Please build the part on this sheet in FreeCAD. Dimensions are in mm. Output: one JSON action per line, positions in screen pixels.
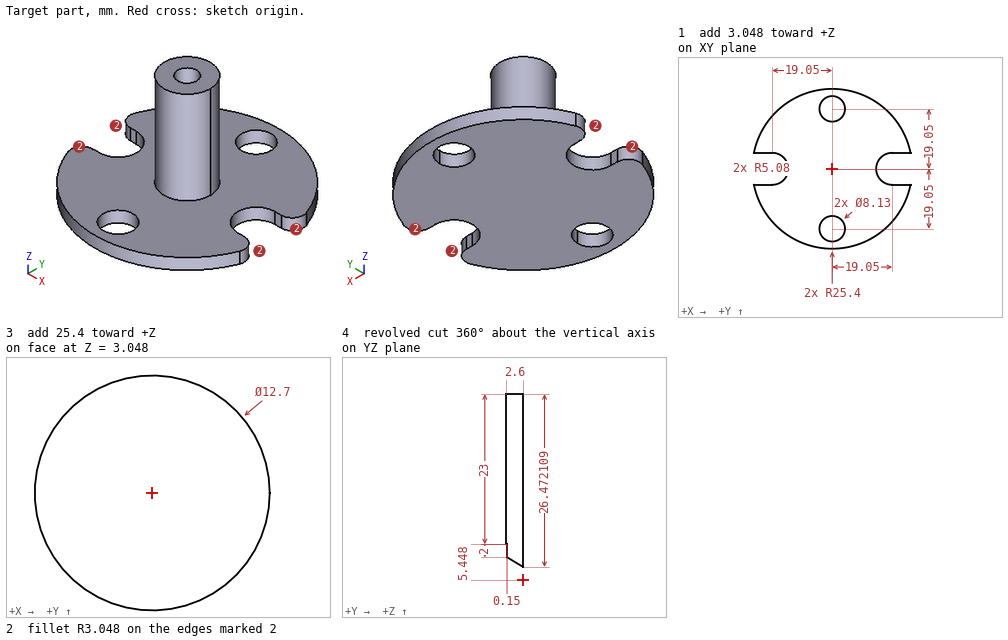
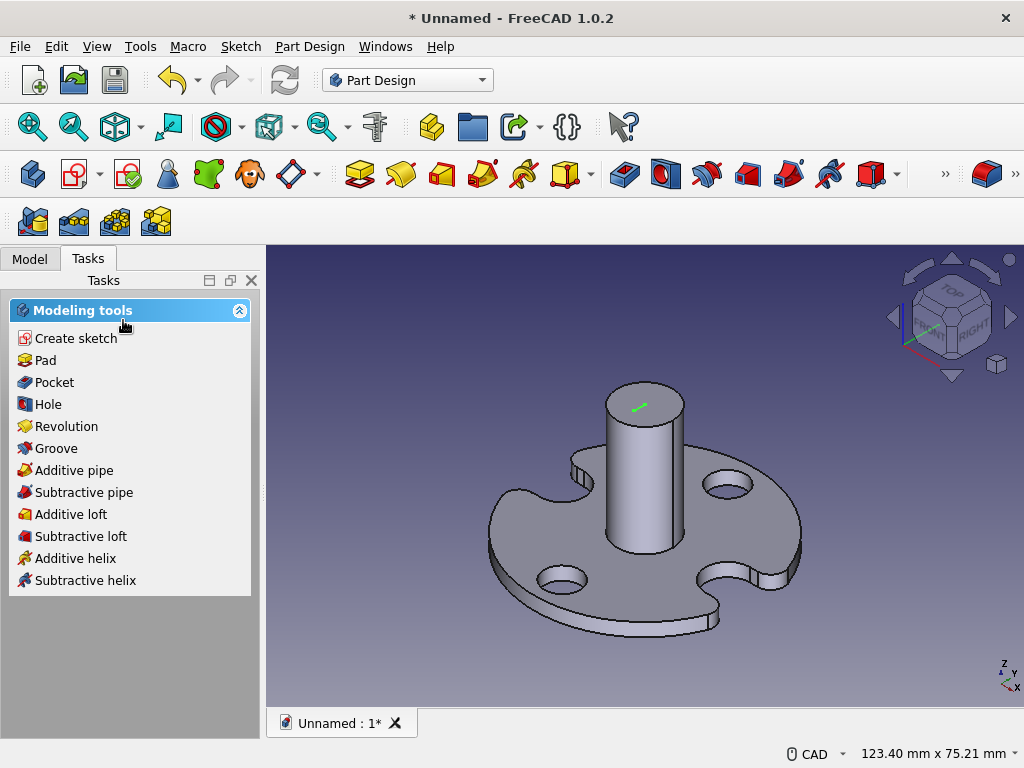
{"action": "left_click", "coordinate": [707, 174]}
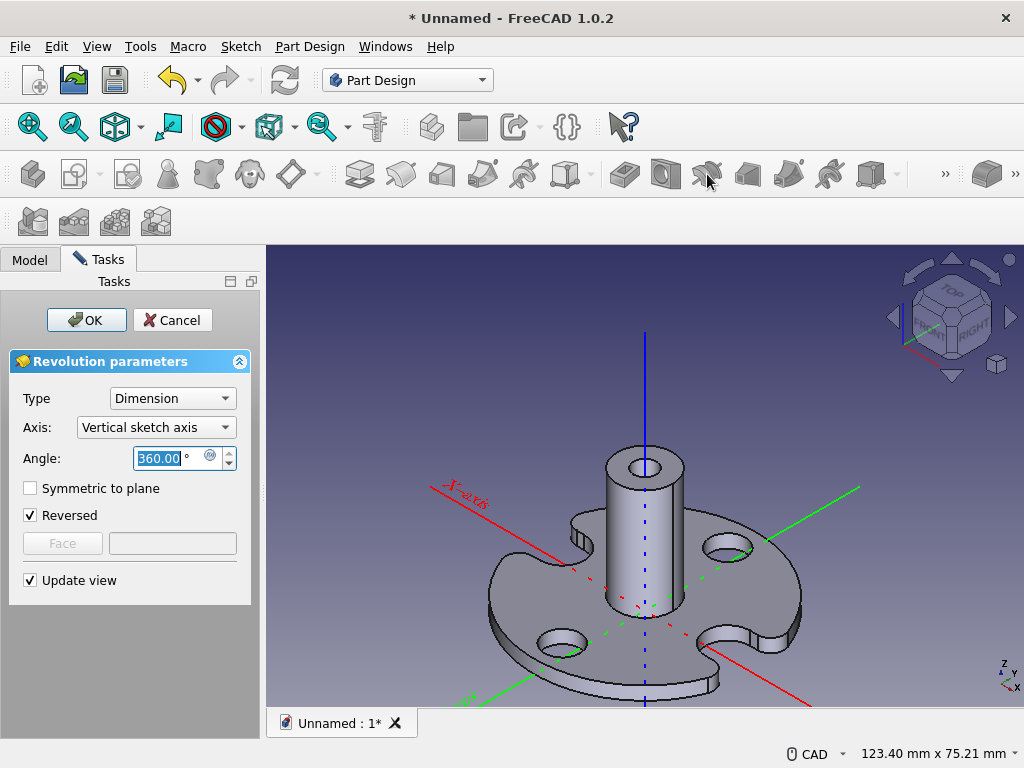
{"action": "left_click", "coordinate": [87, 320]}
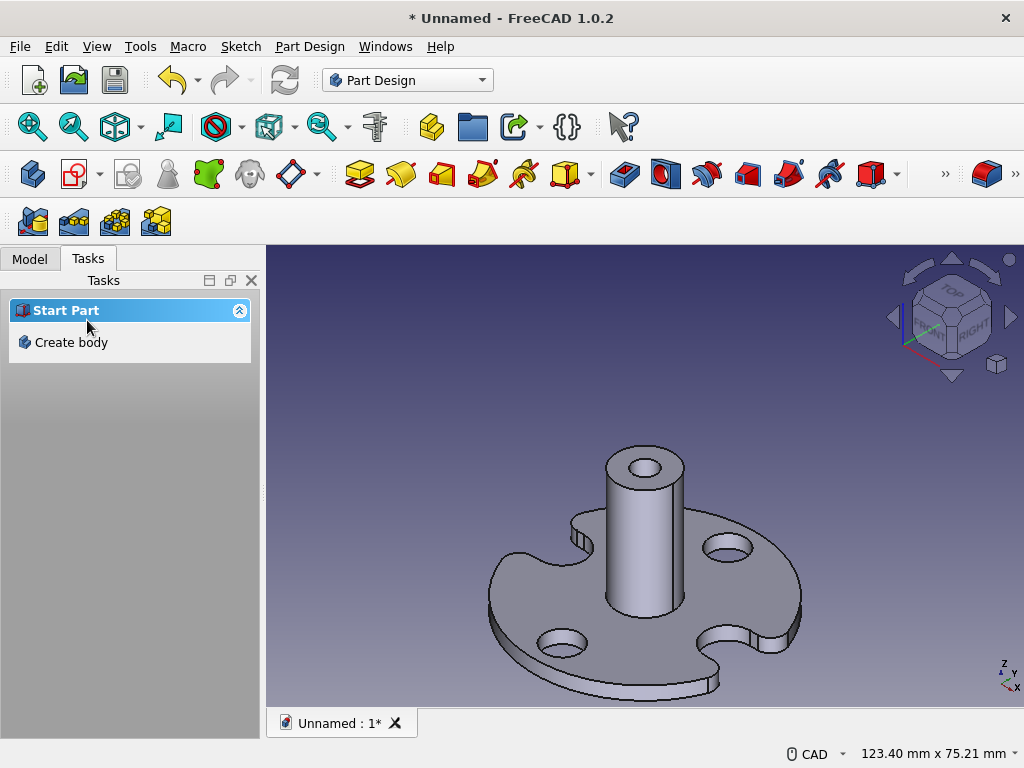
{"action": "left_click", "coordinate": [33, 128]}